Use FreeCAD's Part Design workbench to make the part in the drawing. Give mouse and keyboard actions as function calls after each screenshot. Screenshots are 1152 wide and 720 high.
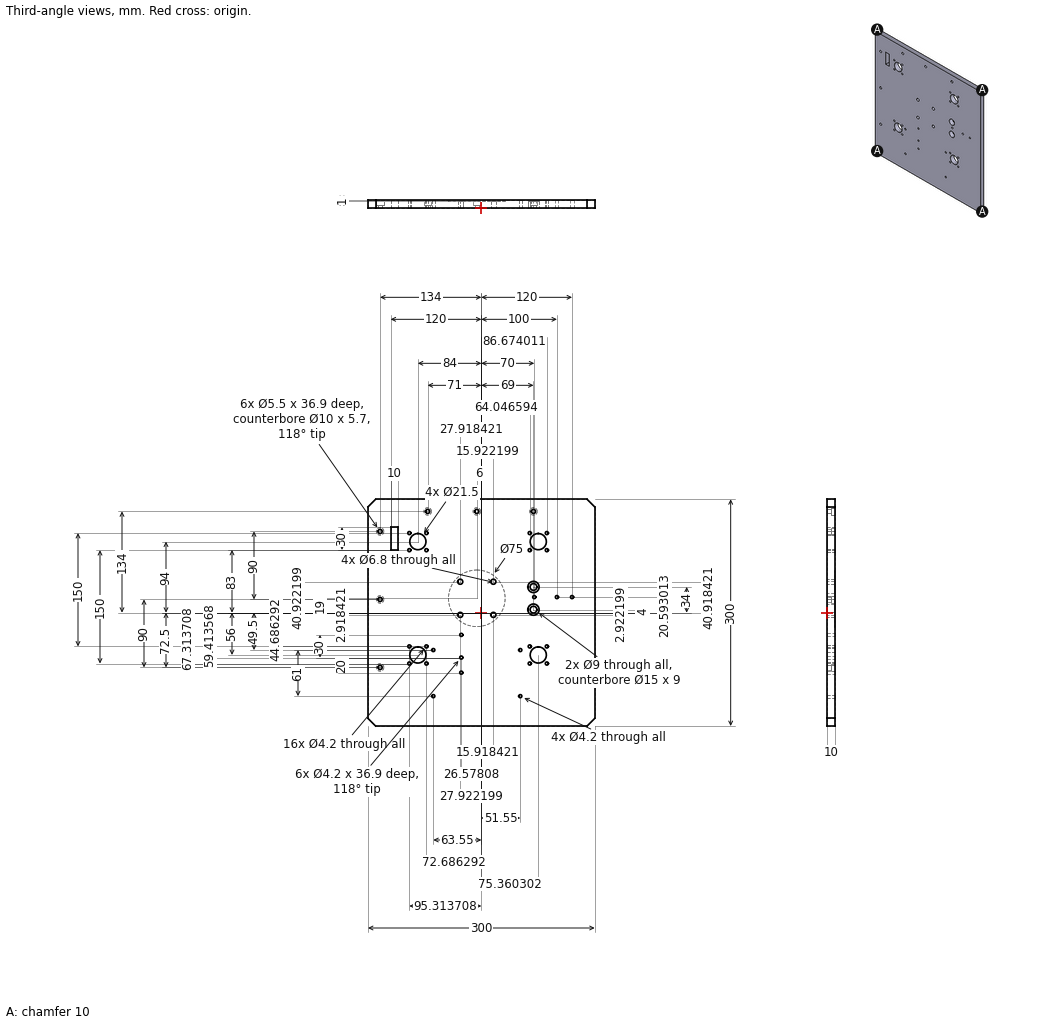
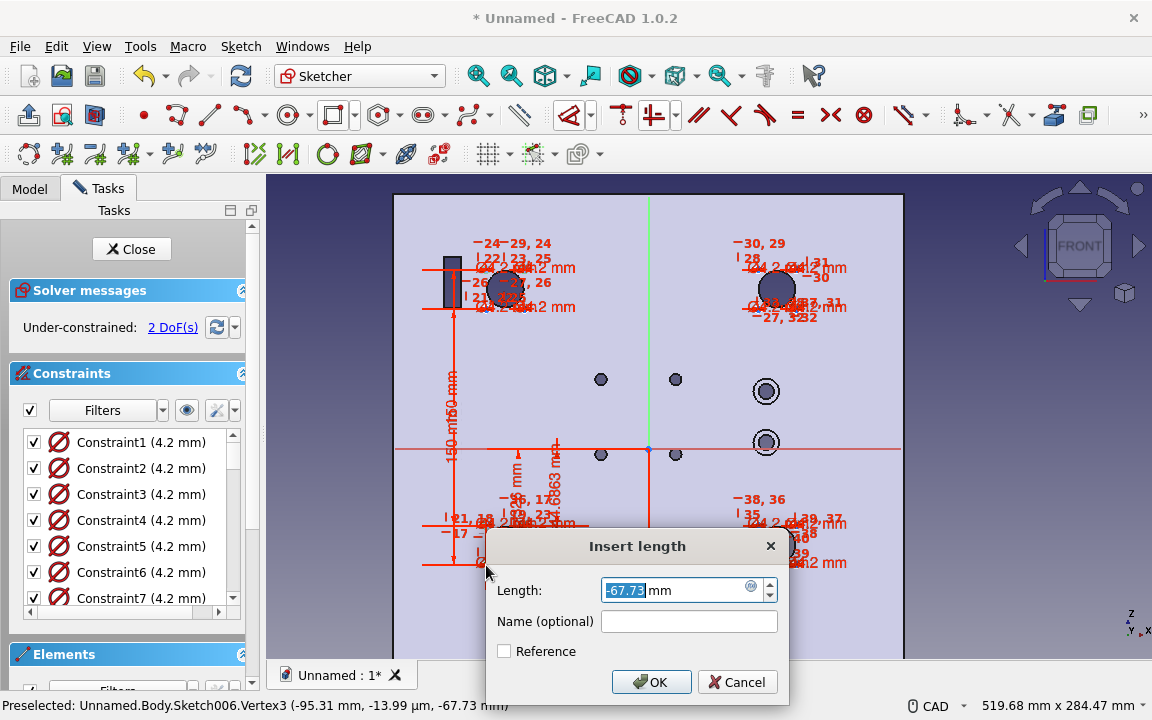
text(-67.313708)
key(Return)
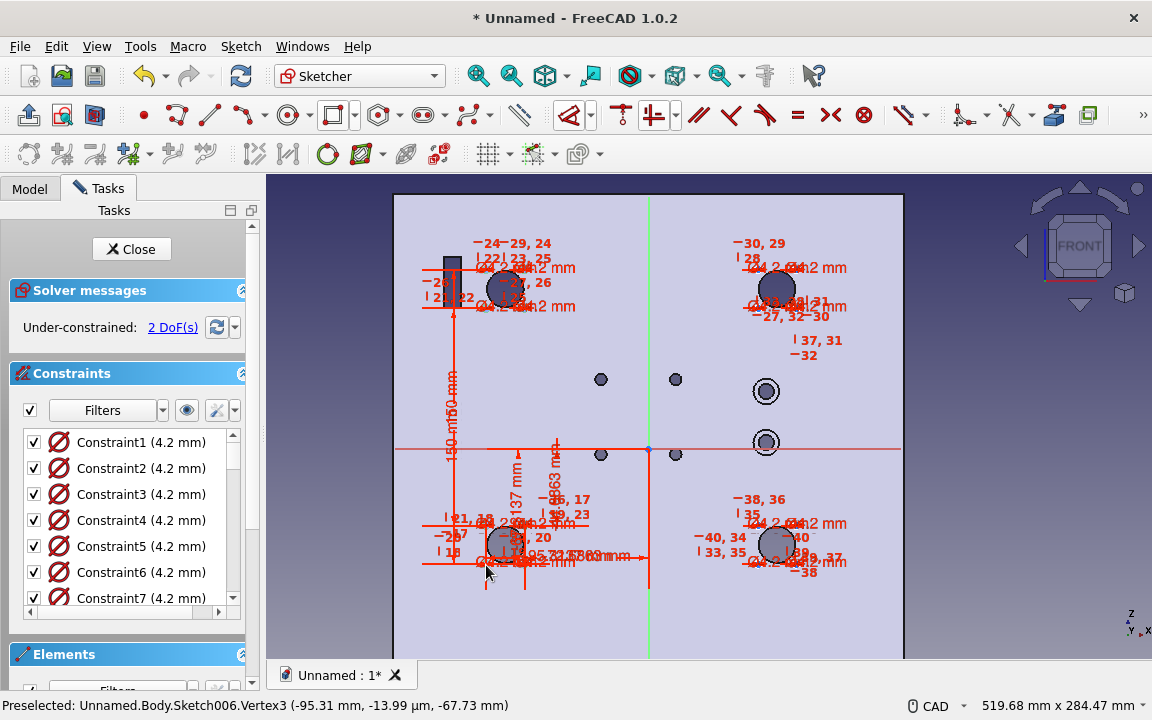
click(758, 308)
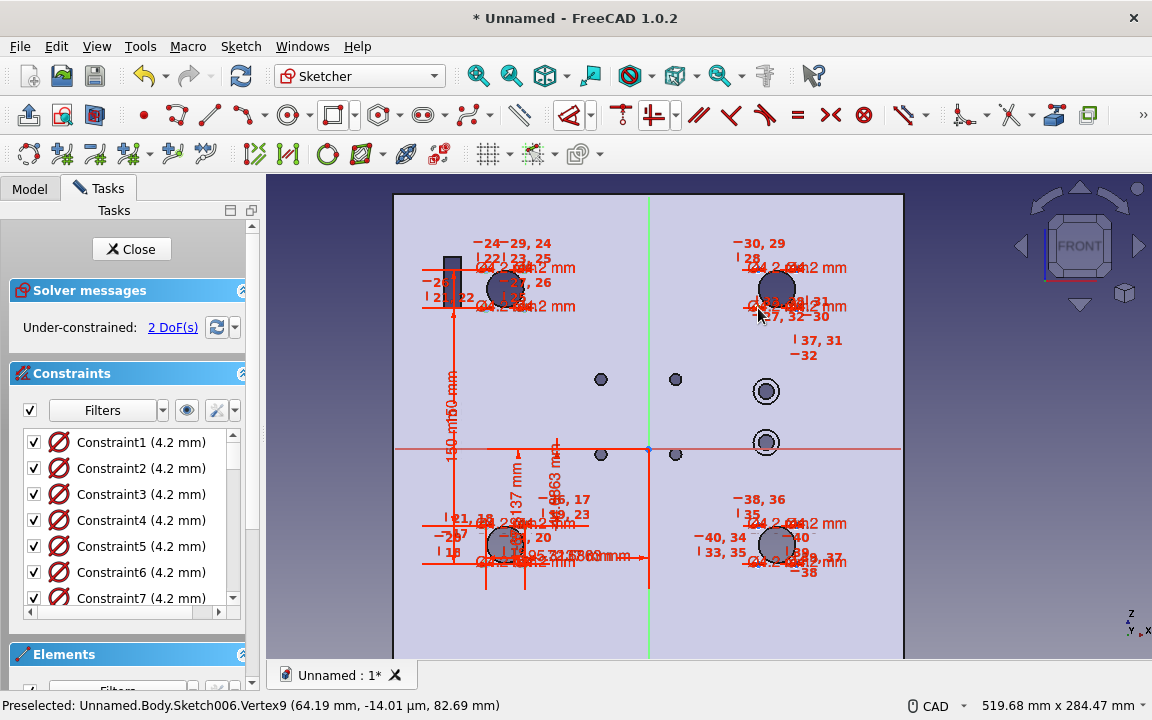
click(590, 116)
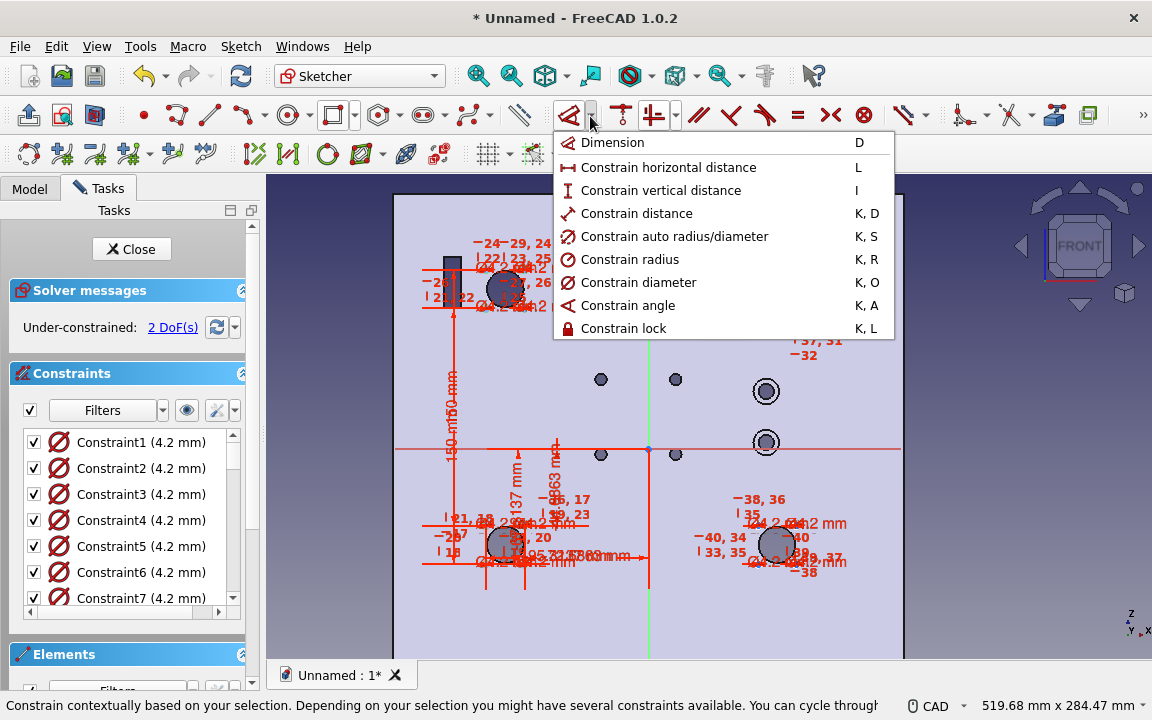
click(724, 168)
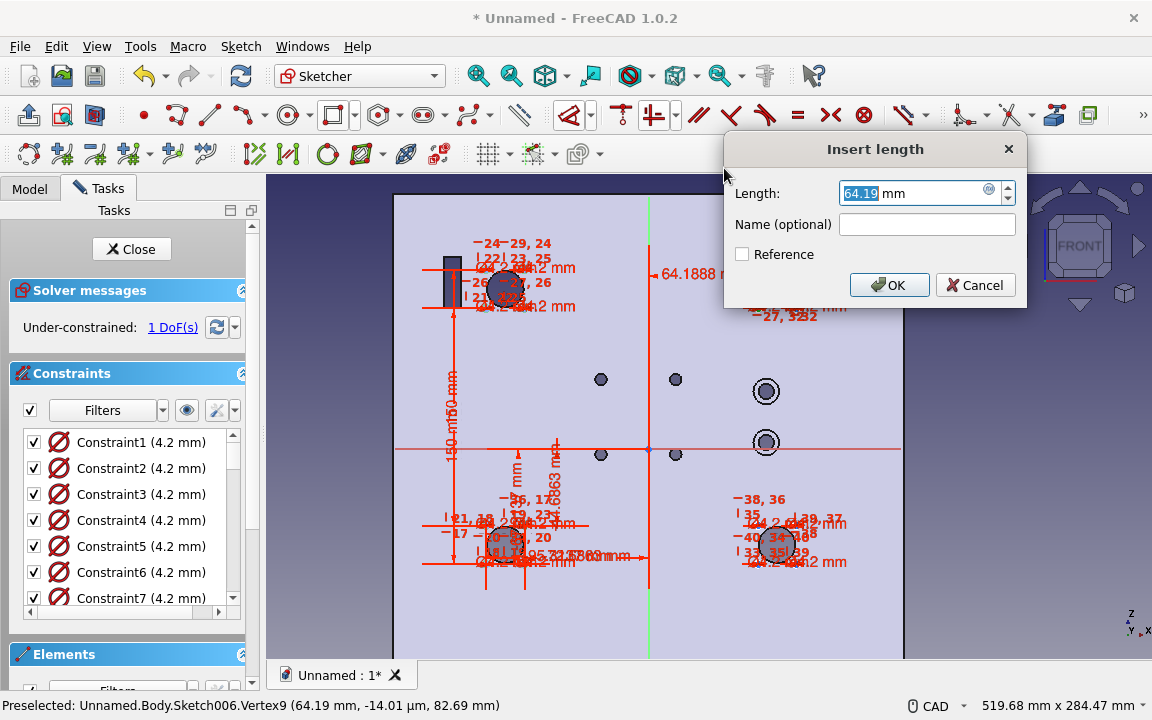
text(64.046594)
key(Return)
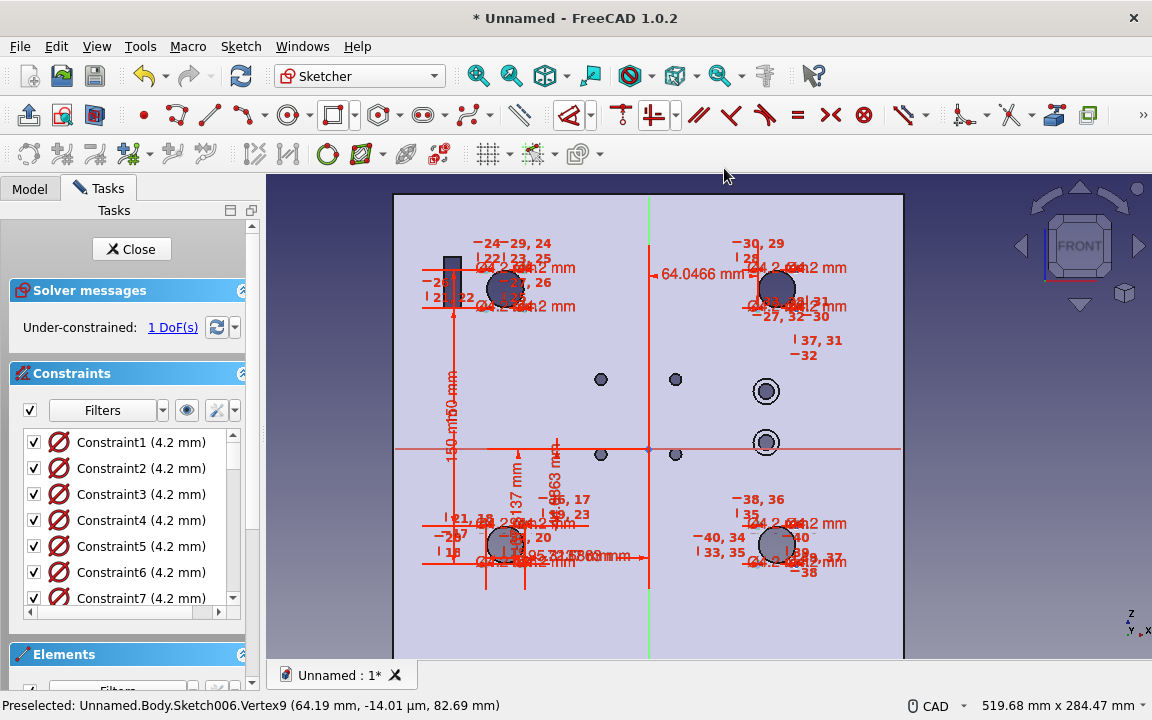
click(796, 270)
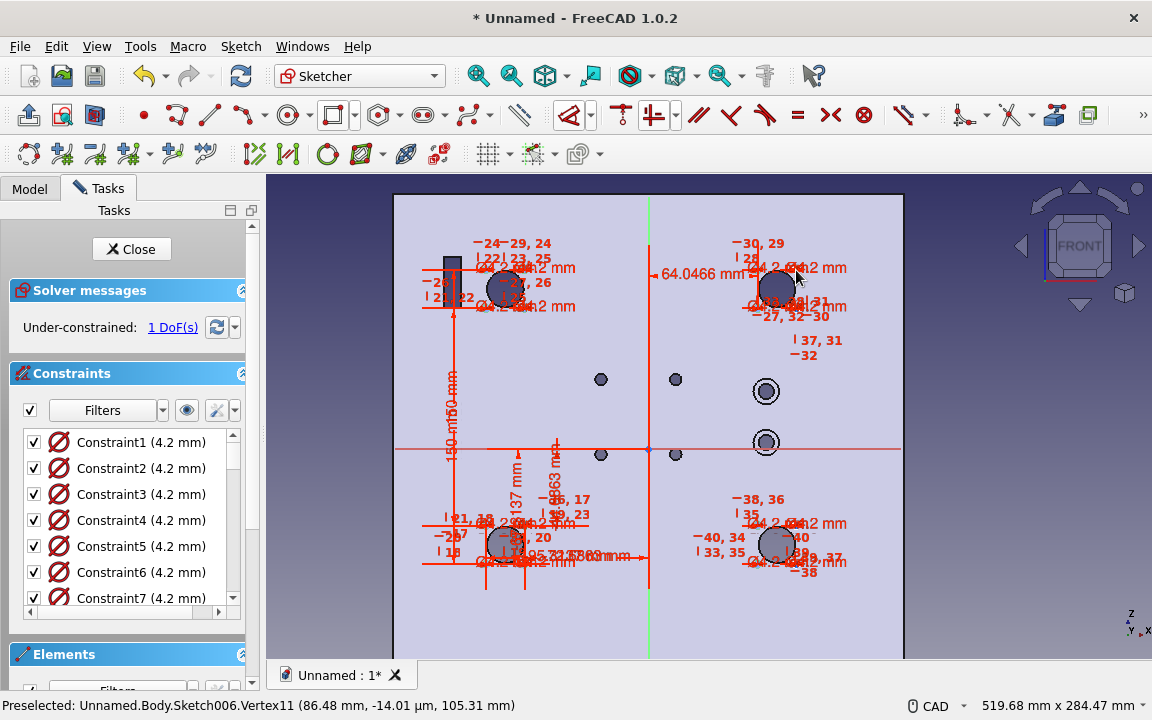
key(l)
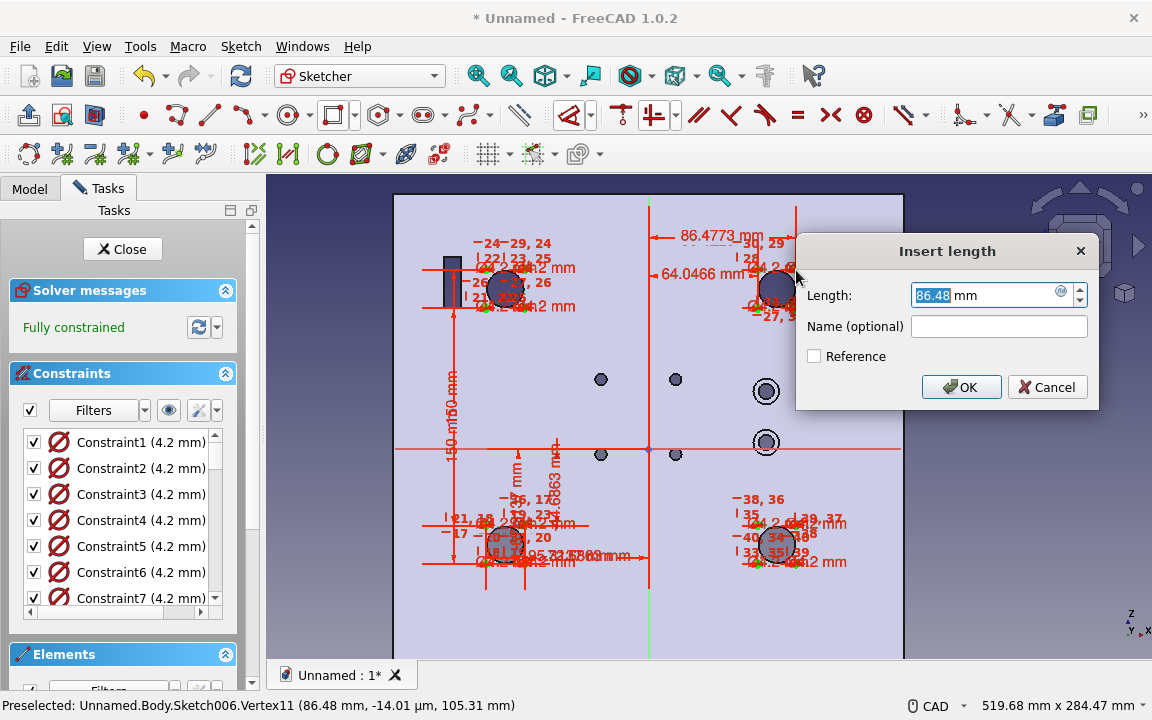
text(86.674011)
key(Return)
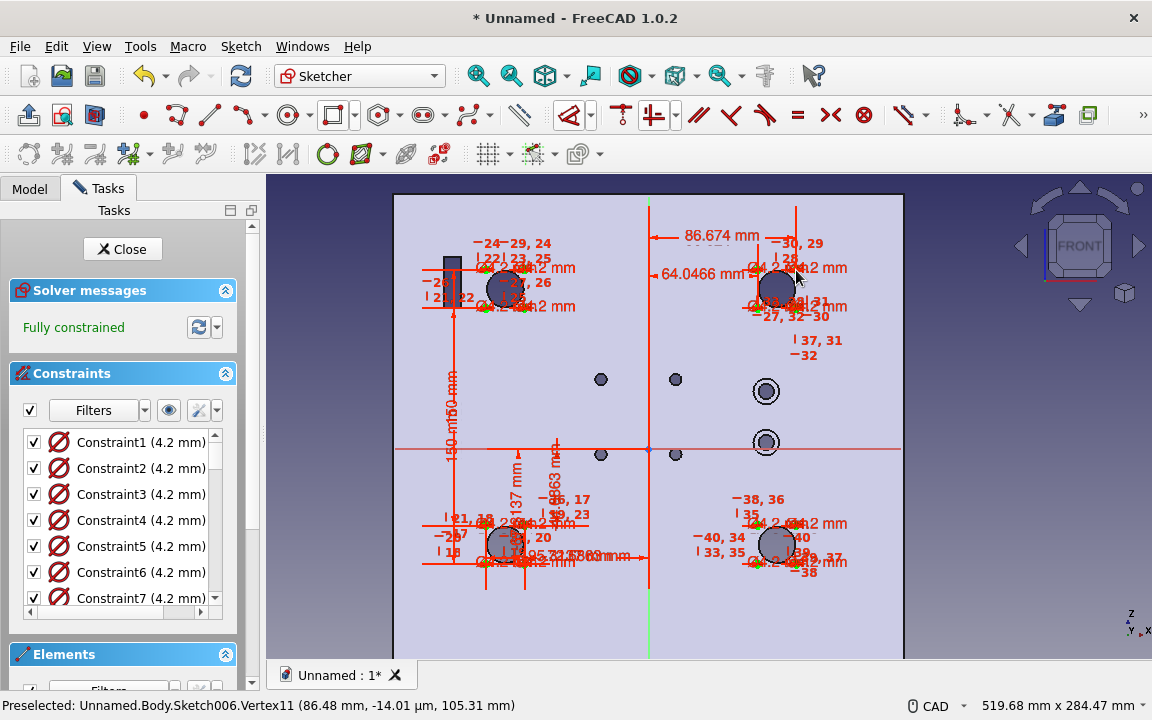
click(123, 249)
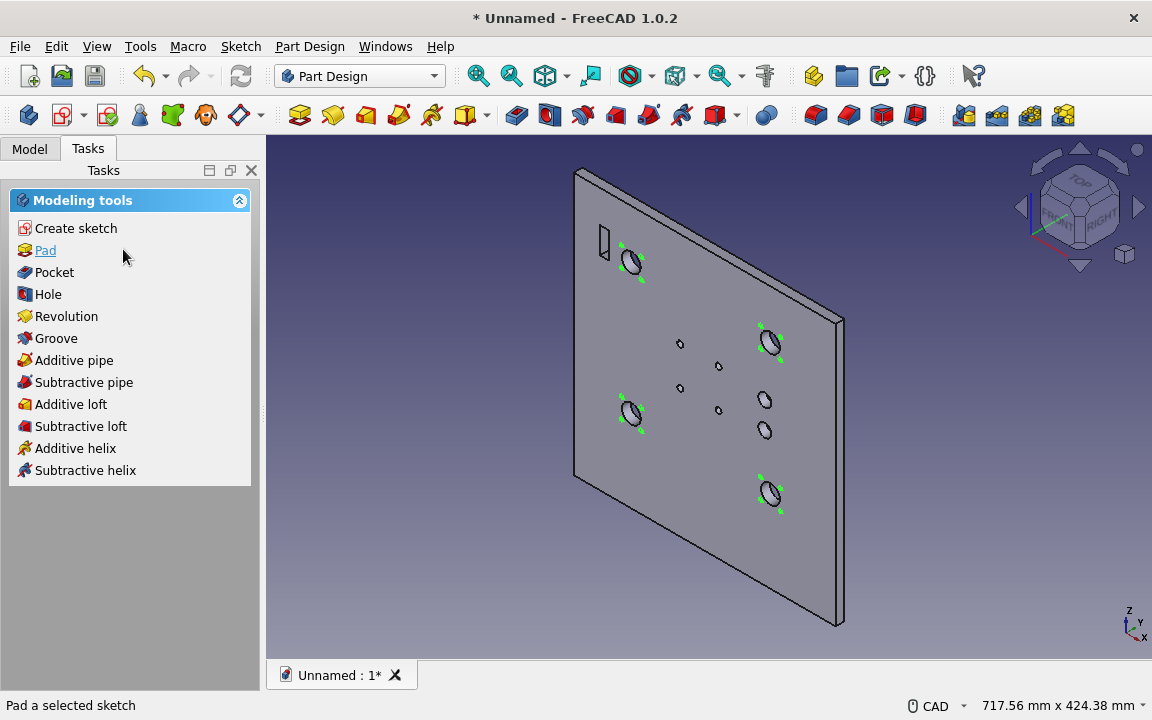
click(550, 116)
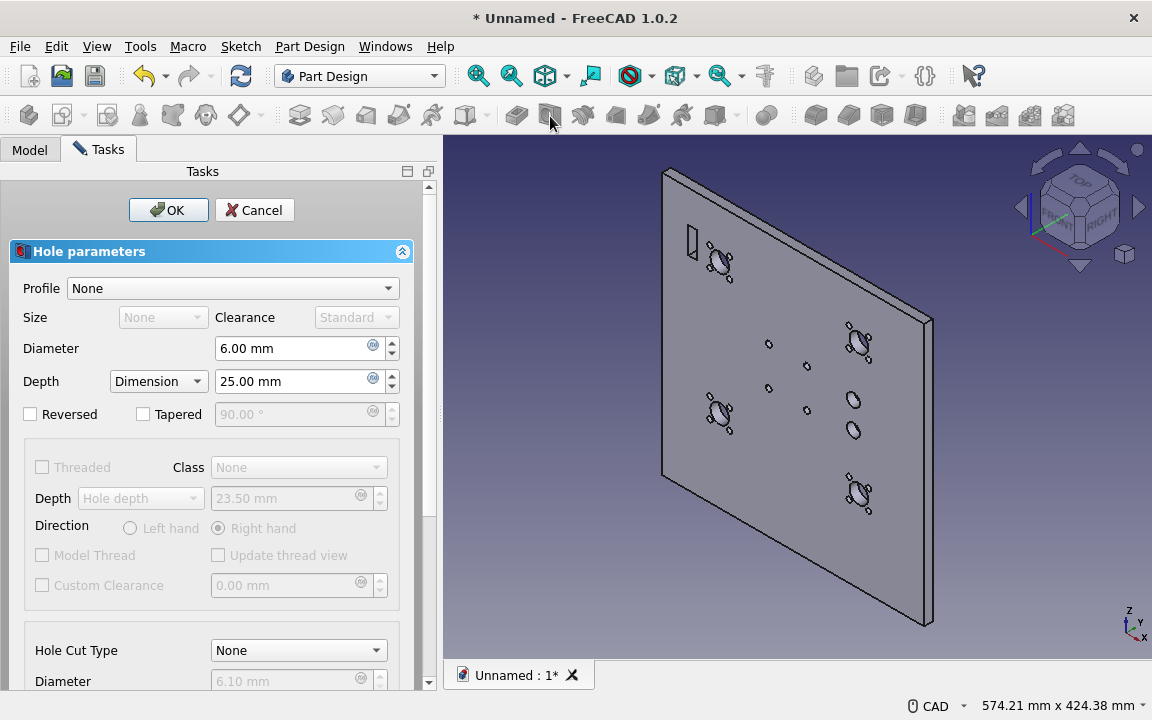
triple_click(300, 348)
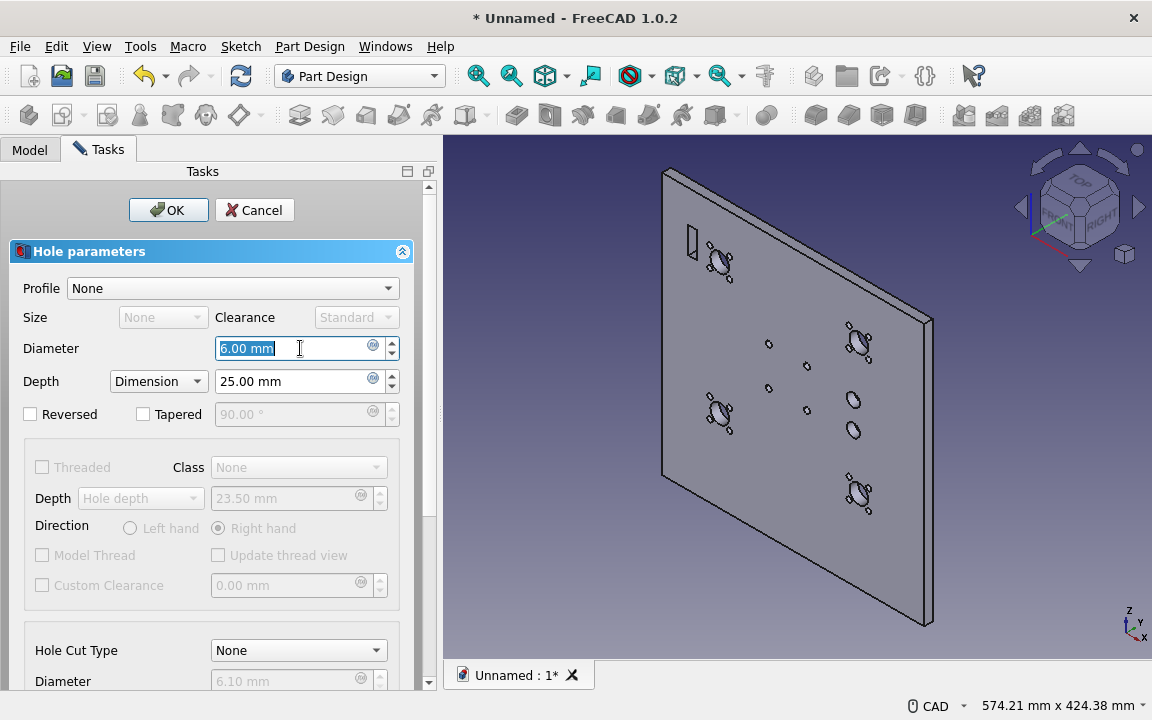
text(4.2)
key(Tab)